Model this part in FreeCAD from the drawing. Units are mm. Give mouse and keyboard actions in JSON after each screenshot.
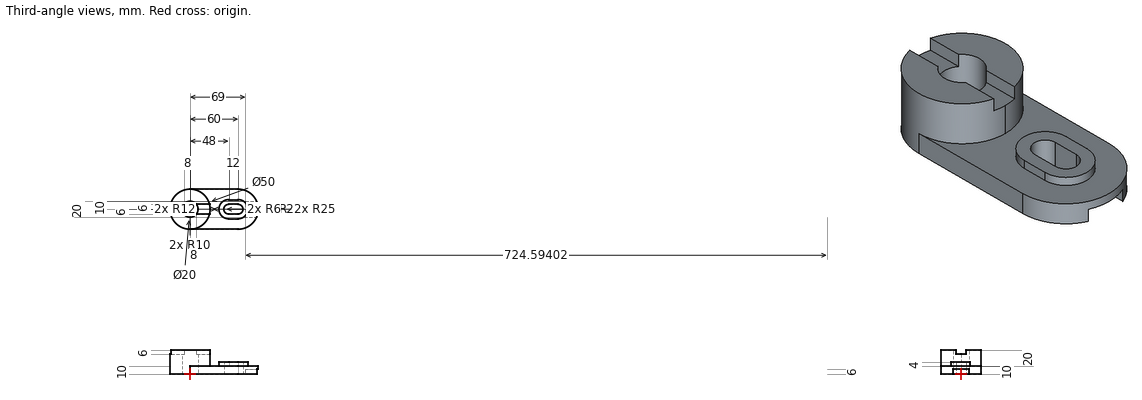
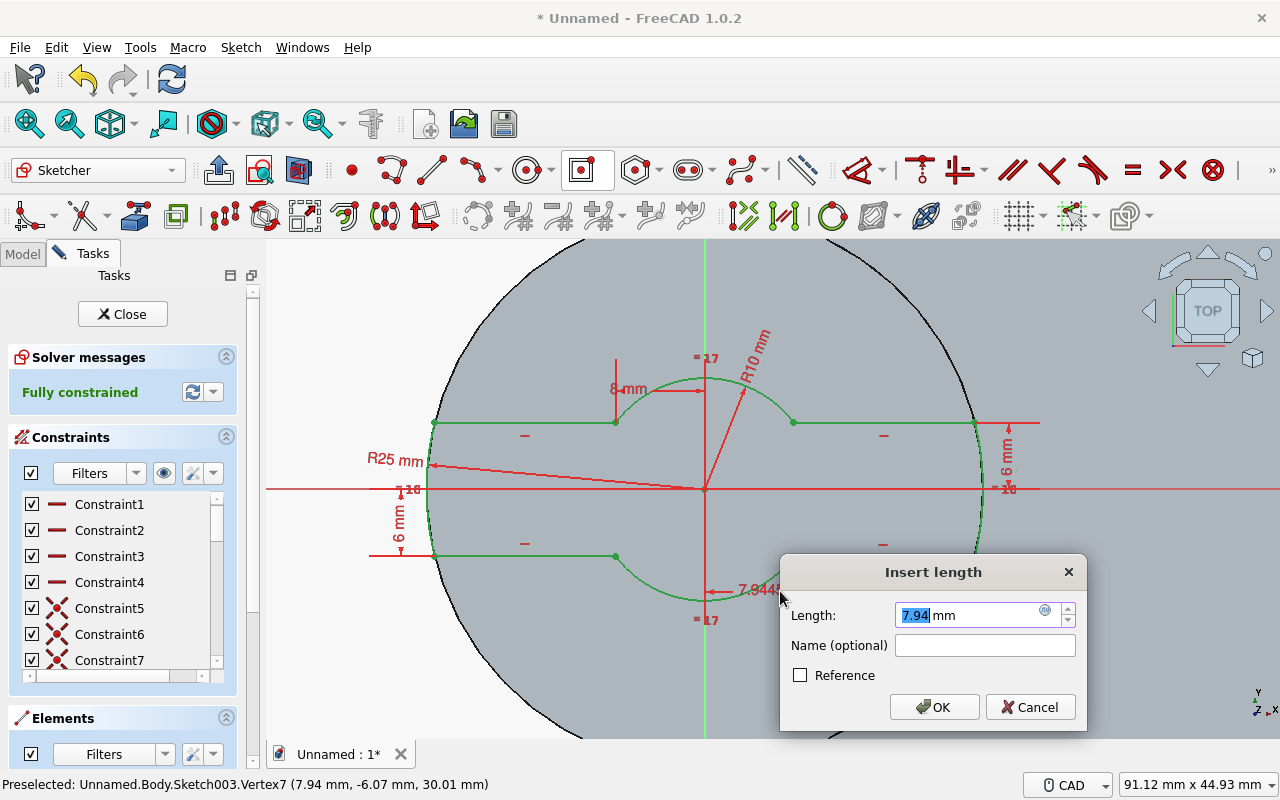
{"action": "type", "text": "8"}
{"action": "key", "text": "Return"}
{"action": "key", "text": "Escape"}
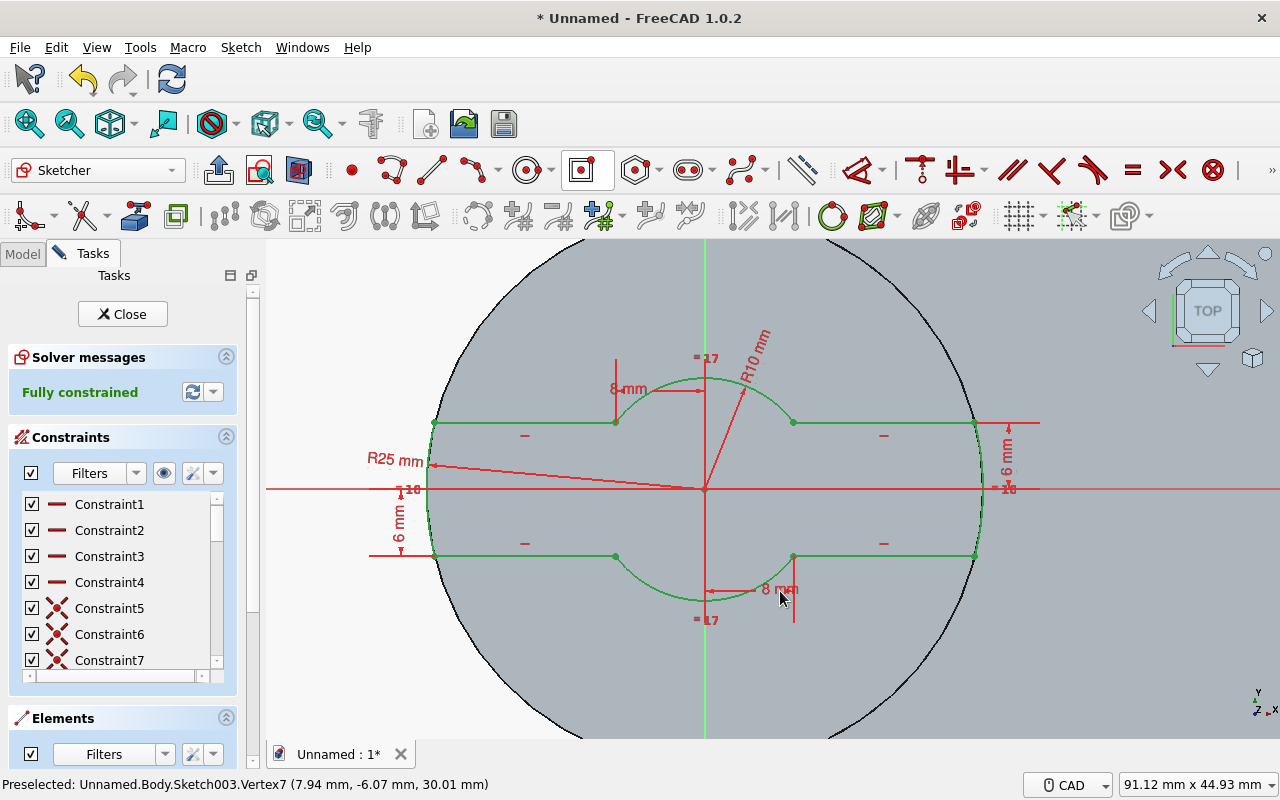
{"action": "left_click", "coordinate": [123, 314]}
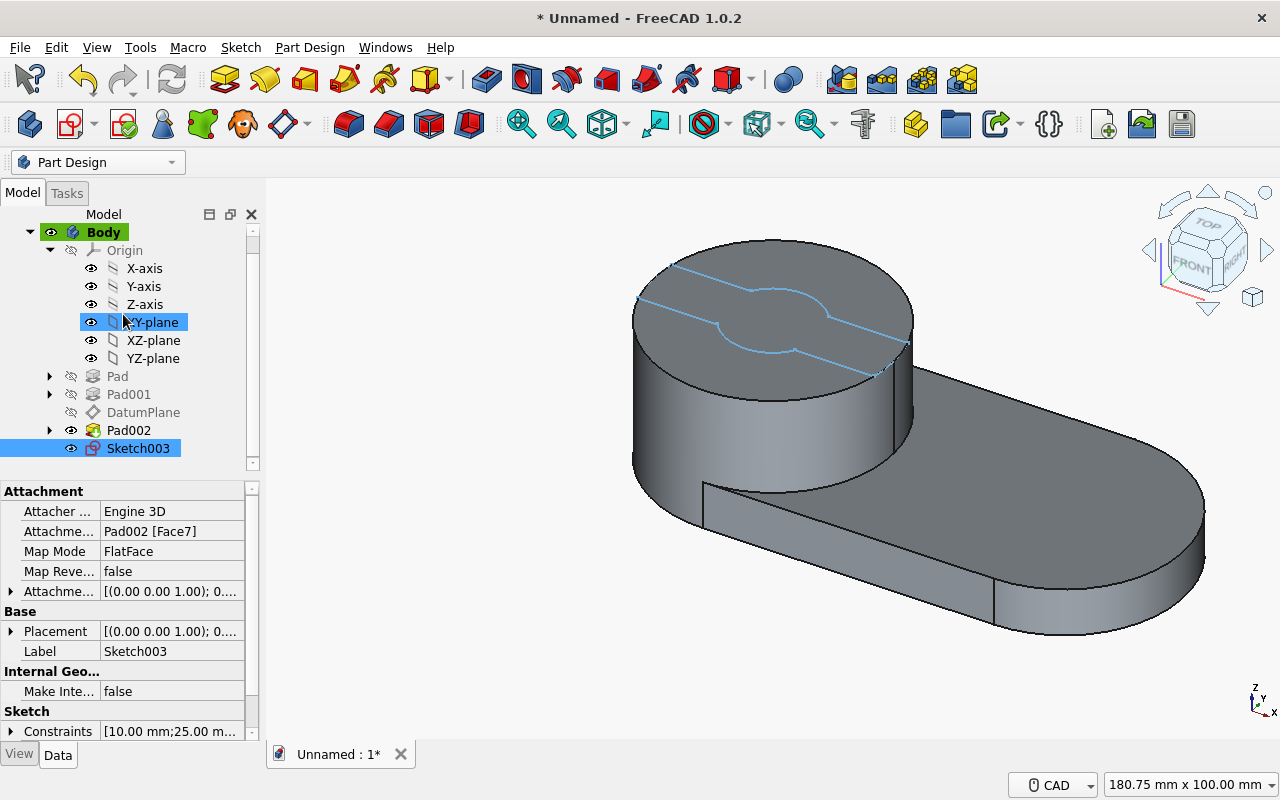
{"action": "left_click", "coordinate": [488, 80]}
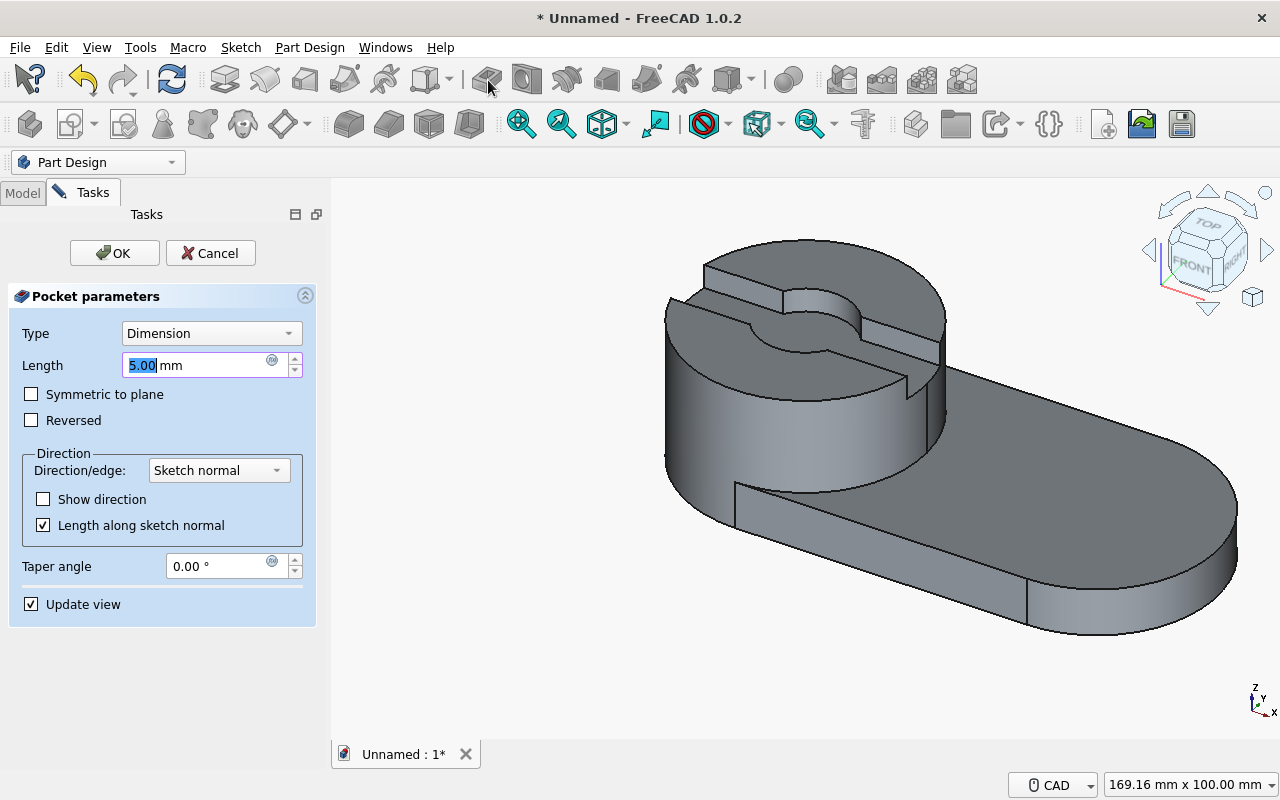
{"action": "type", "text": "6"}
{"action": "key", "text": "Tab"}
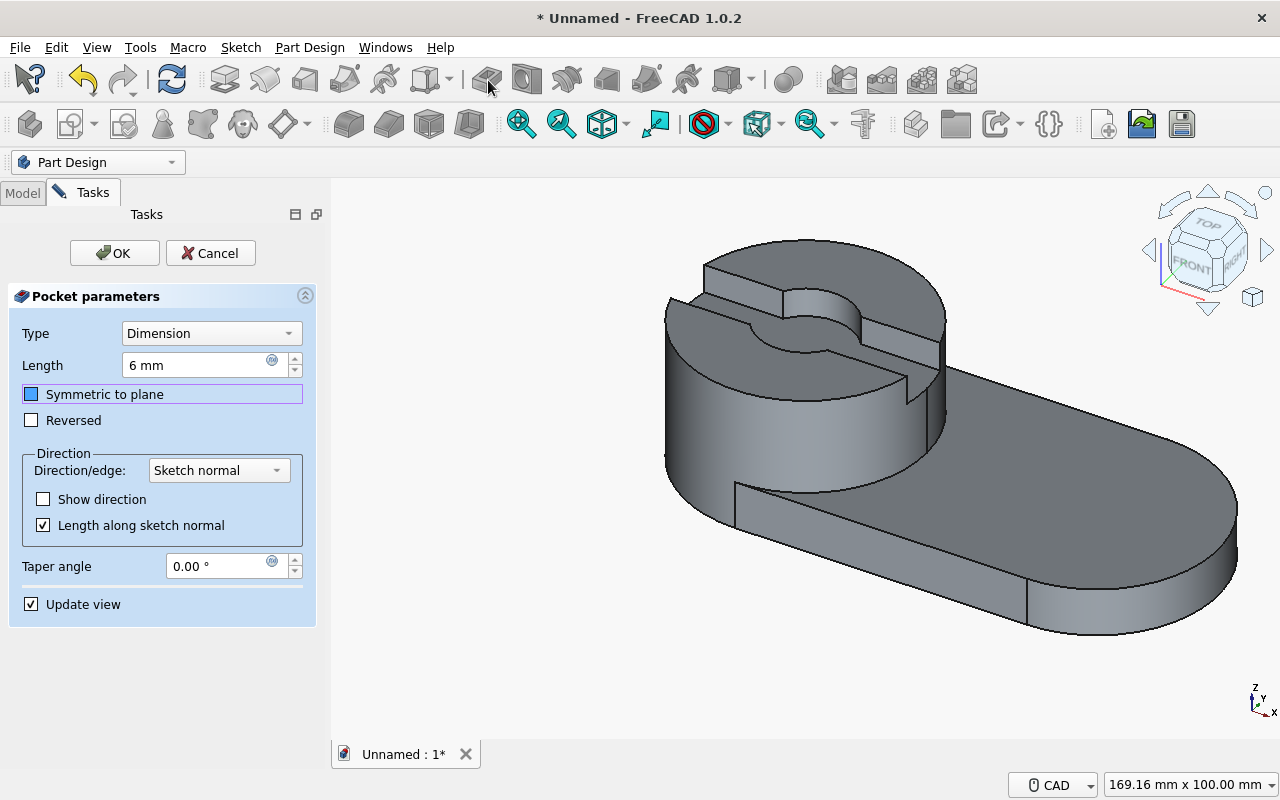
{"action": "left_click", "coordinate": [115, 253]}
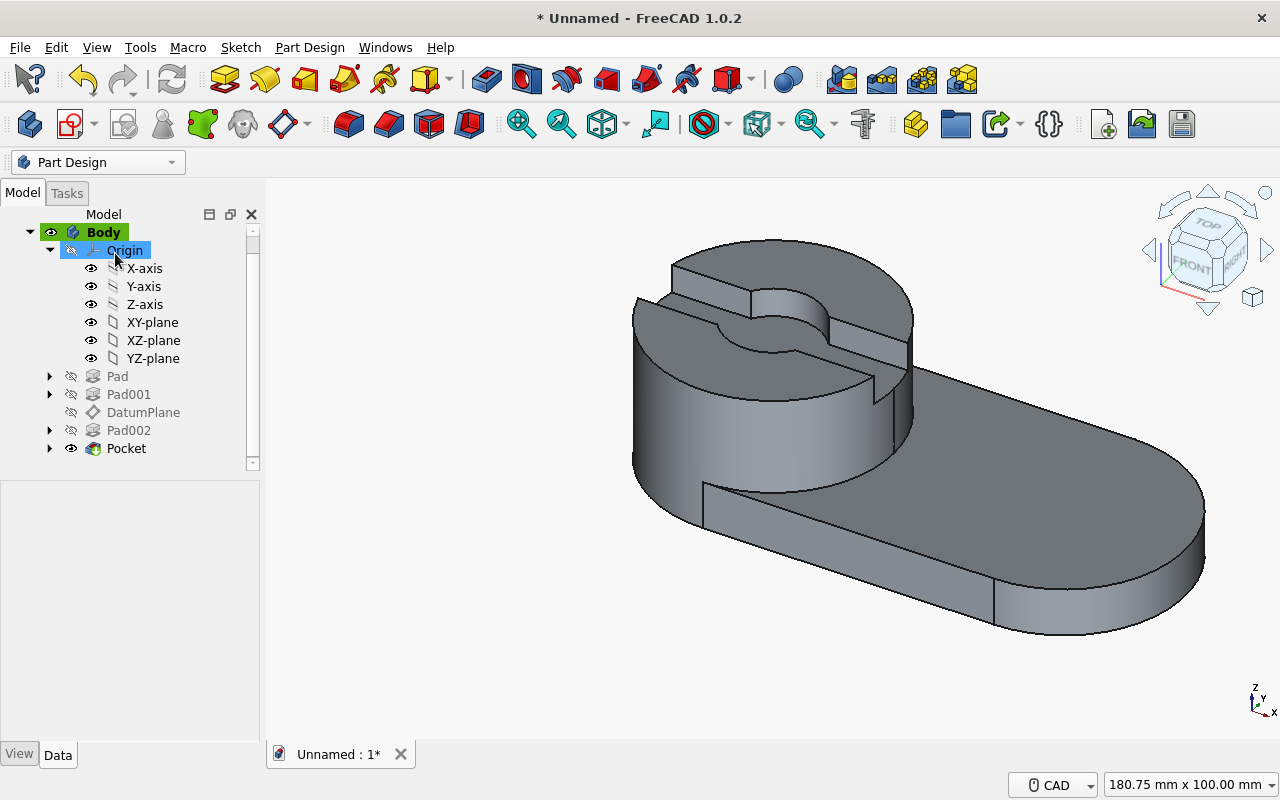
{"action": "left_click", "coordinate": [781, 339]}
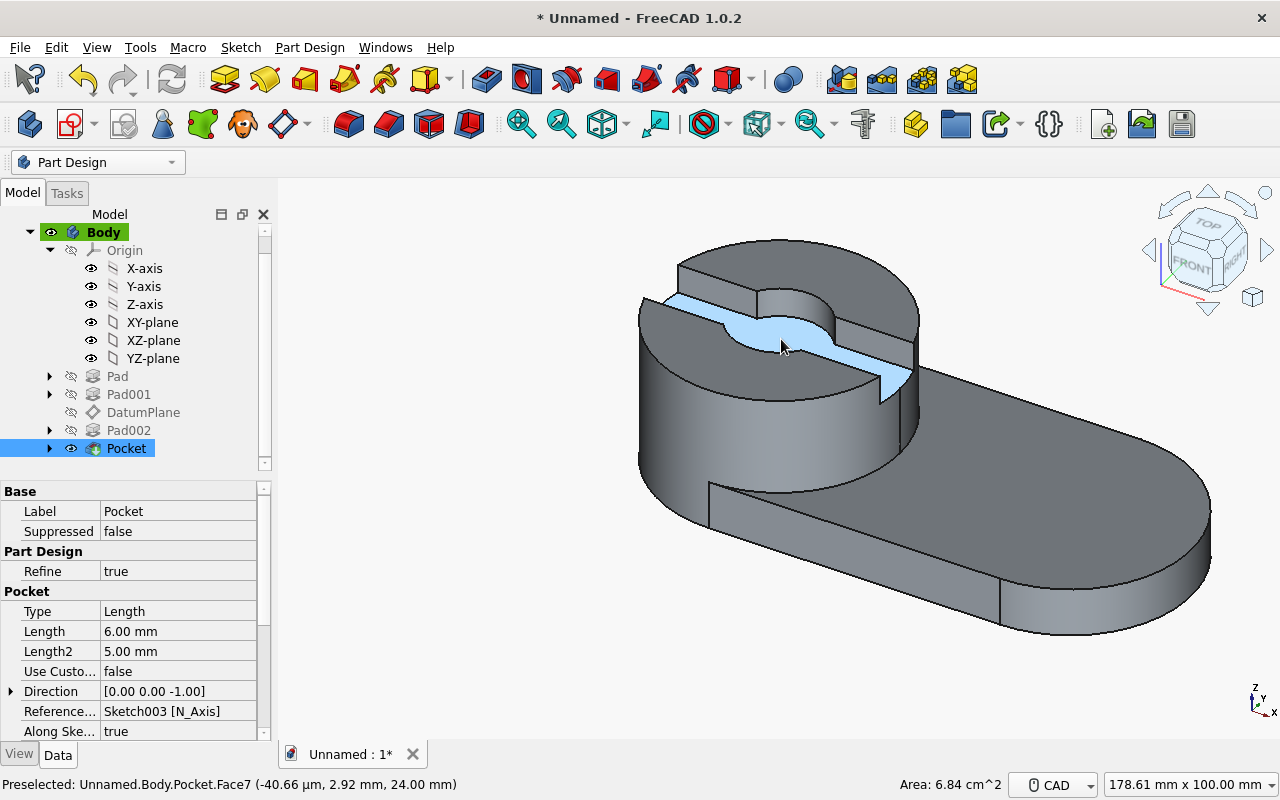
{"action": "left_click", "coordinate": [70, 124]}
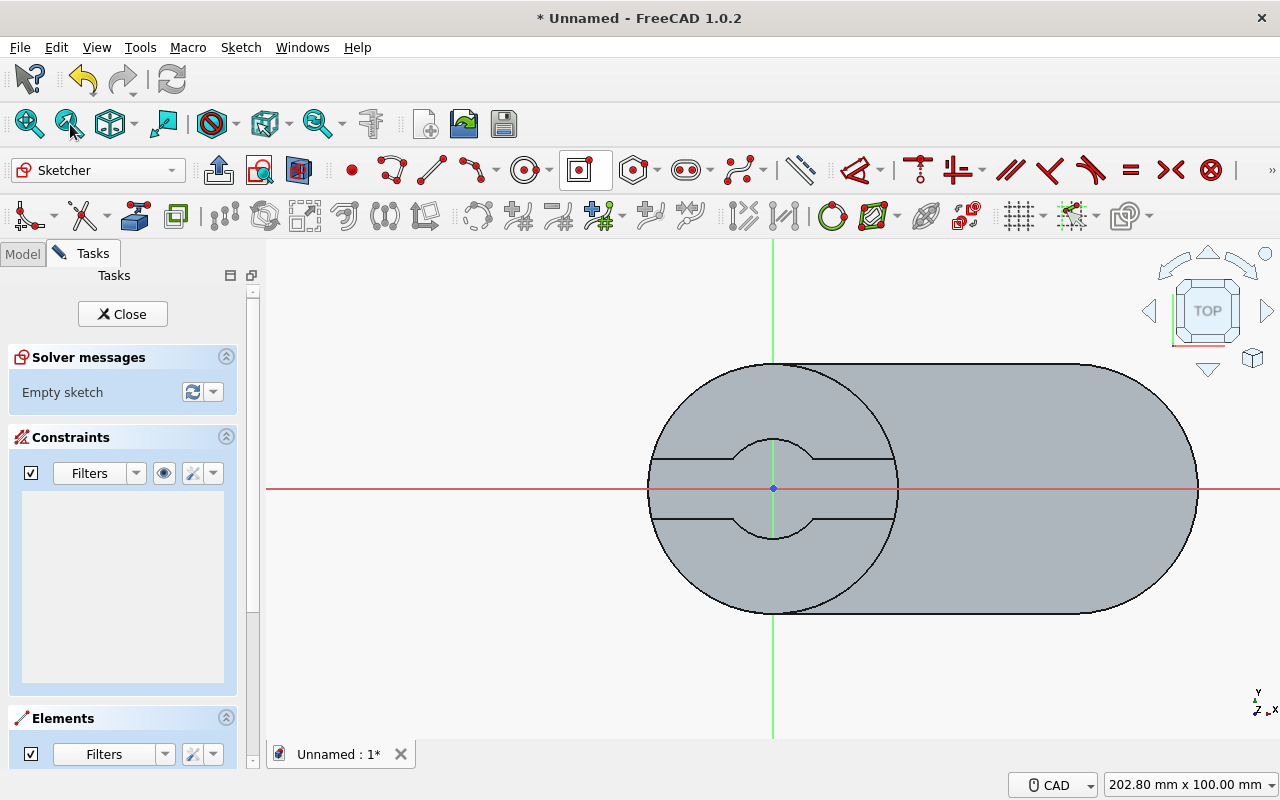
{"action": "left_click", "coordinate": [300, 170]}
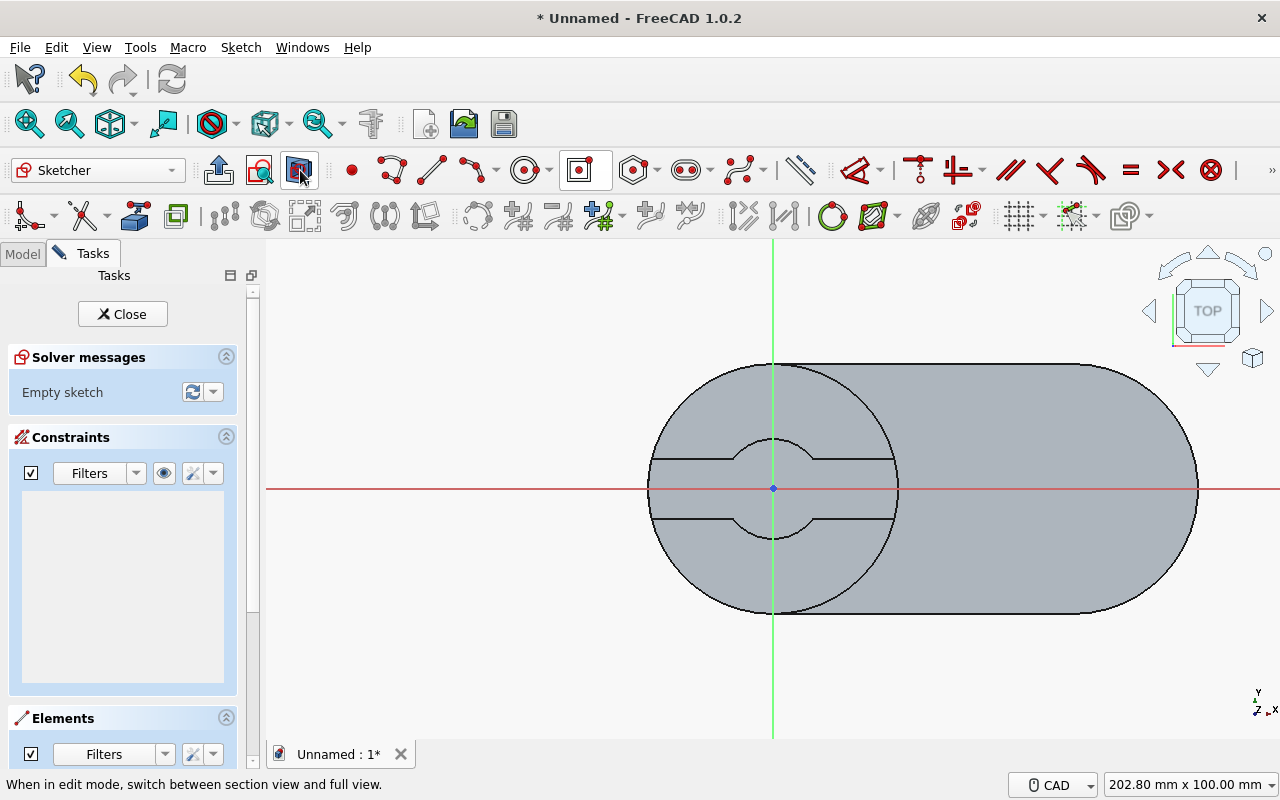
{"action": "scroll", "coordinate": [803, 489], "scroll_direction": "up", "scroll_amount": 6}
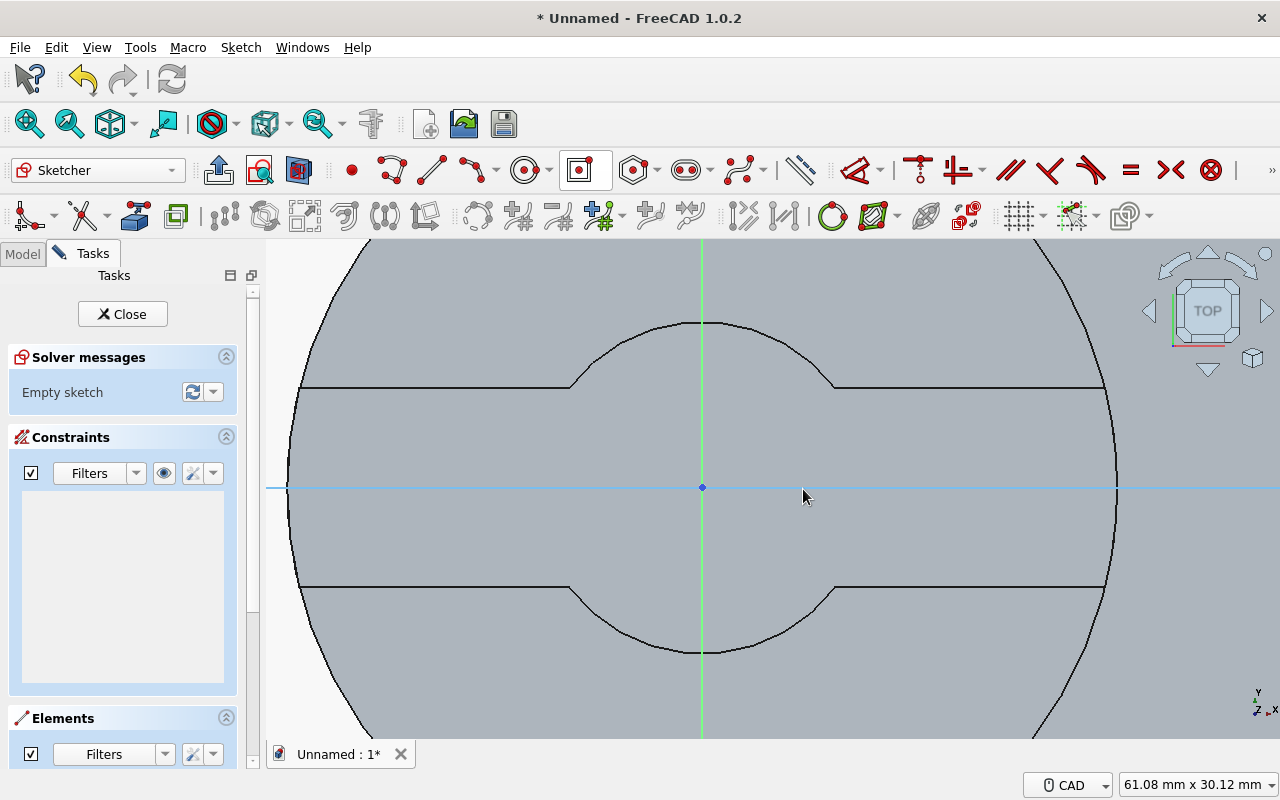
{"action": "left_click", "coordinate": [526, 170]}